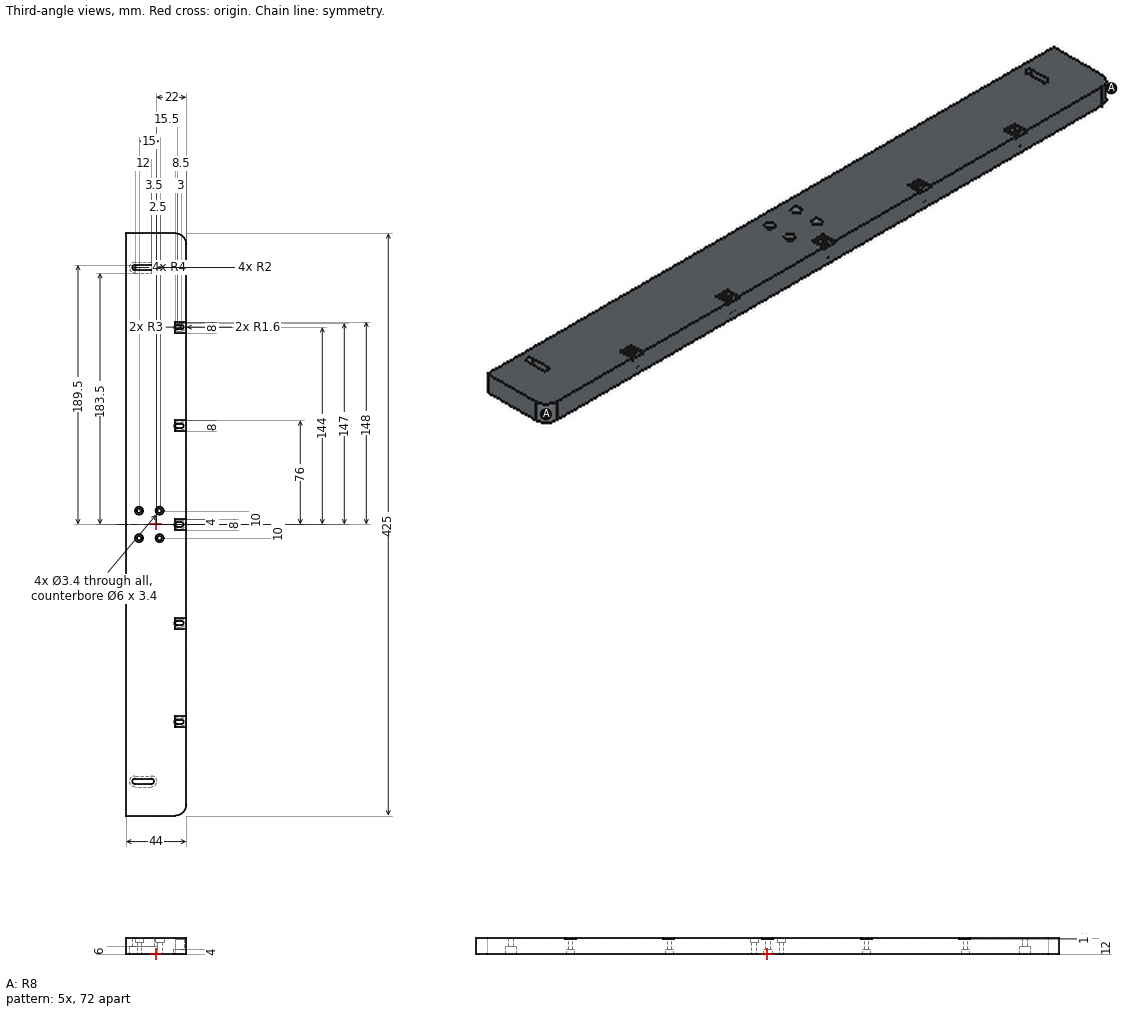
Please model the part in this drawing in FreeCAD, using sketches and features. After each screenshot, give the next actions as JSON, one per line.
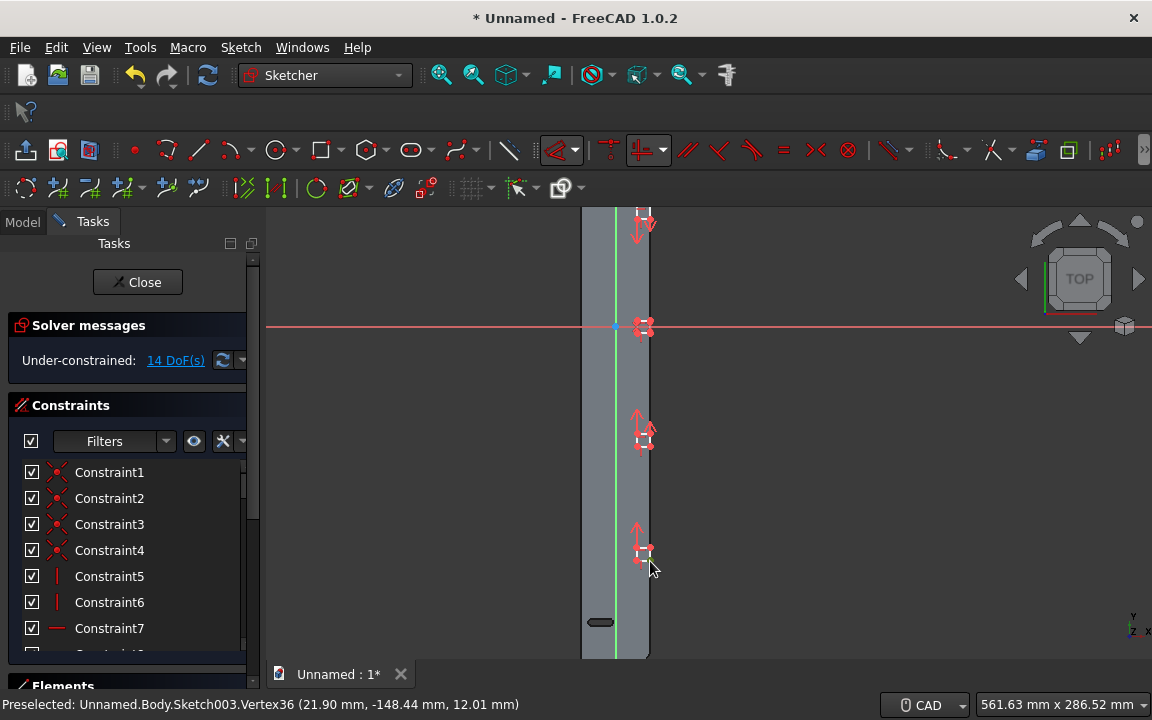
{"action": "left_click", "coordinate": [344, 327]}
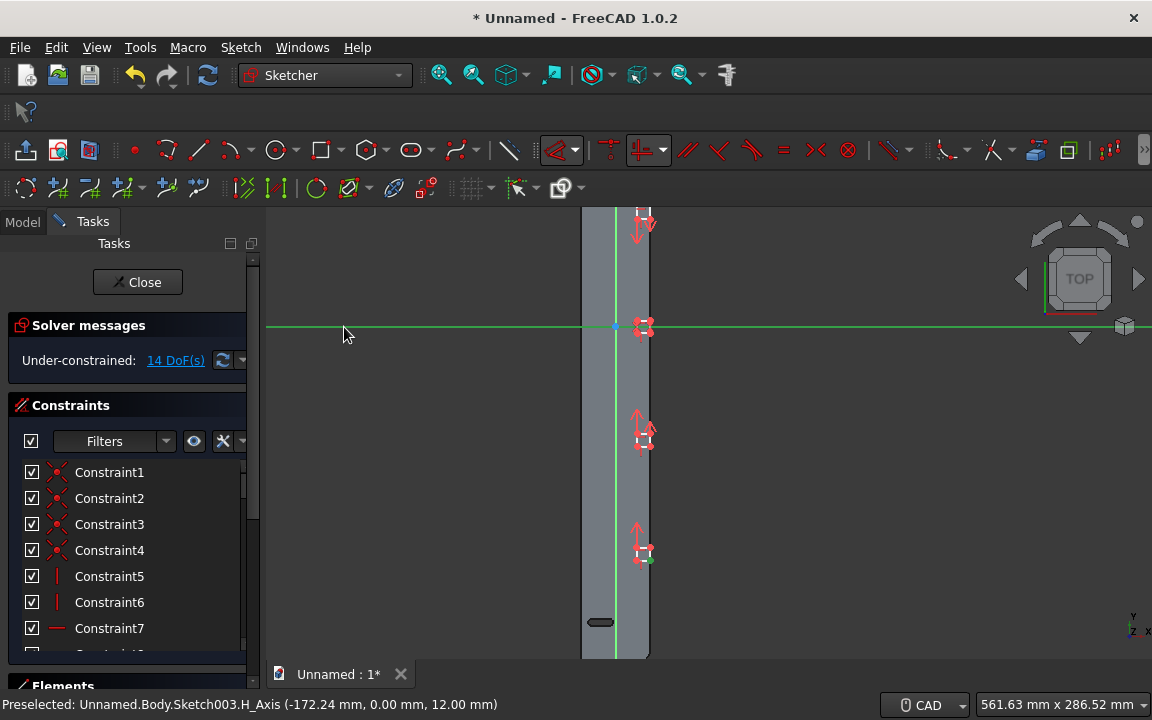
{"action": "key", "text": "s"}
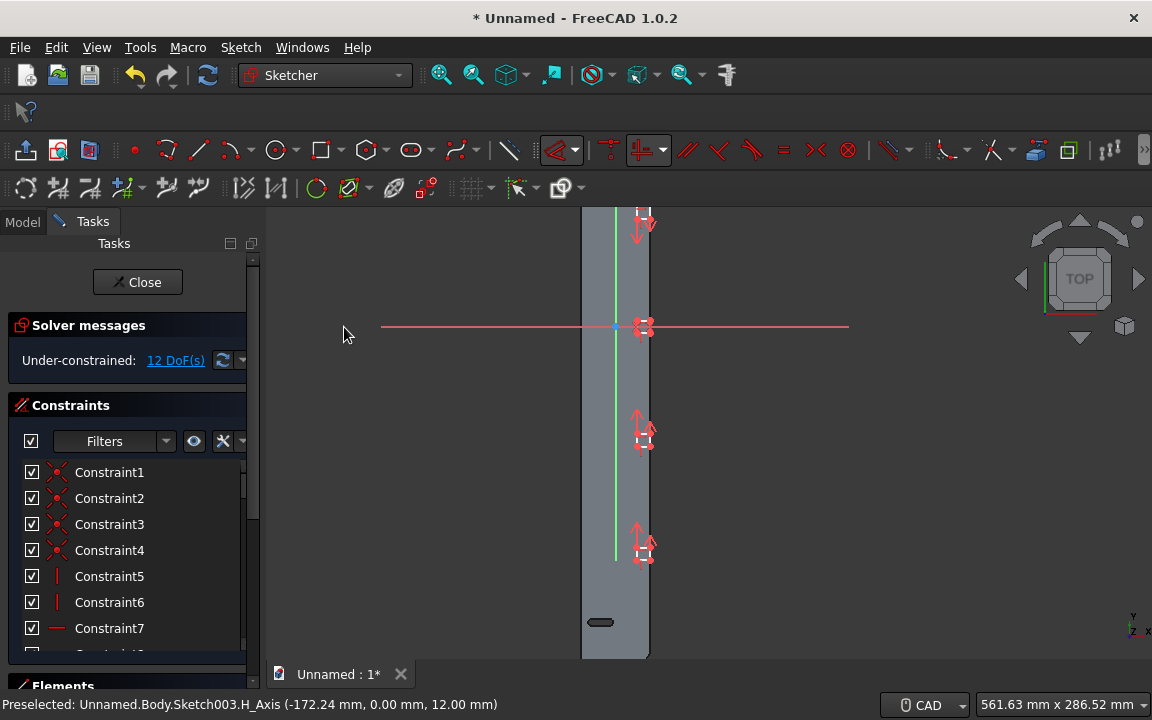
{"action": "scroll", "coordinate": [650, 562], "scroll_direction": "down", "scroll_amount": 3}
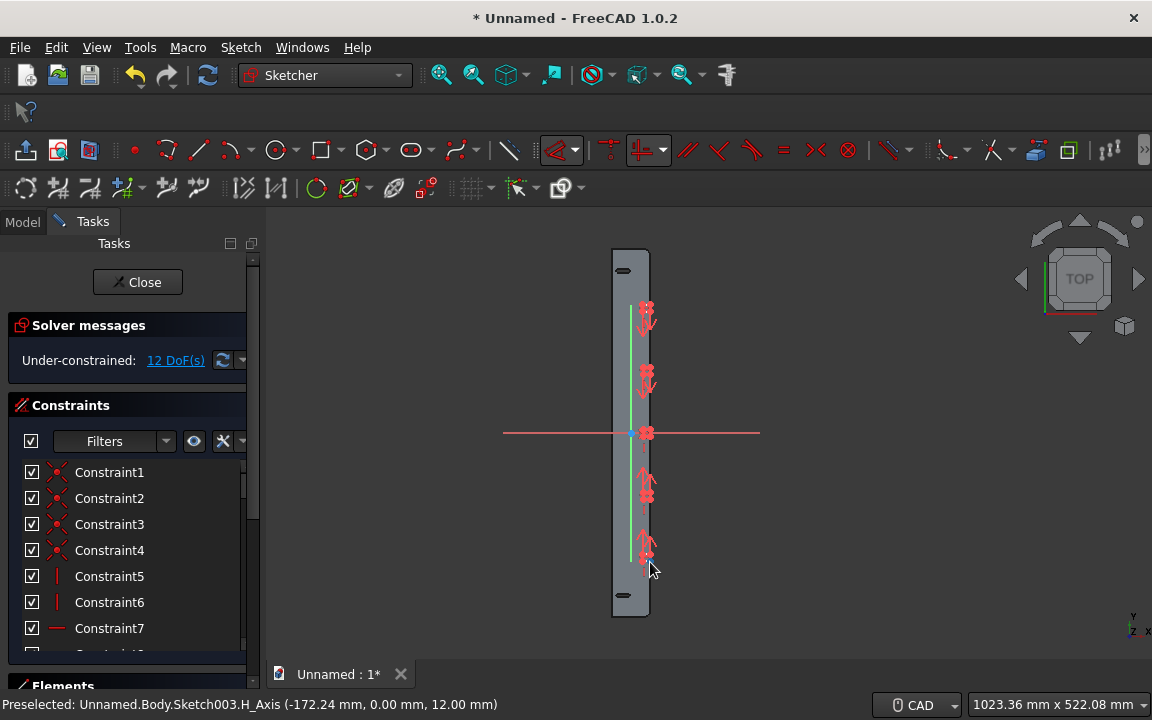
{"action": "scroll", "coordinate": [643, 308], "scroll_direction": "up", "scroll_amount": 9}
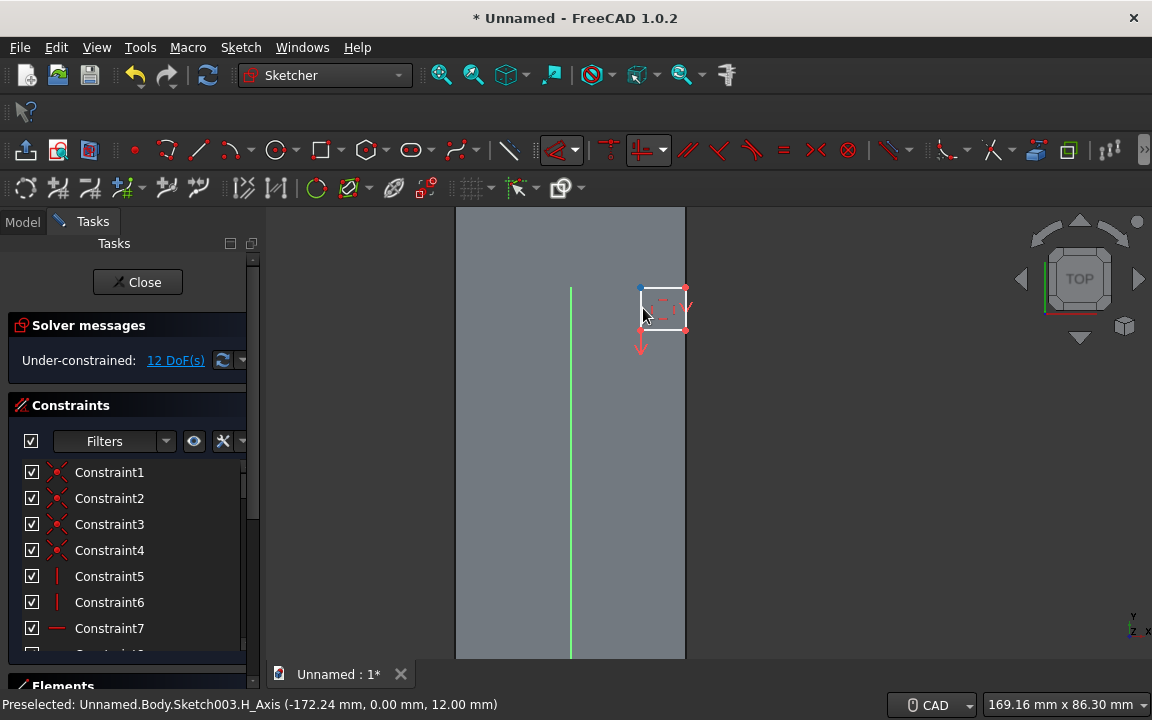
{"action": "left_click", "coordinate": [641, 309]}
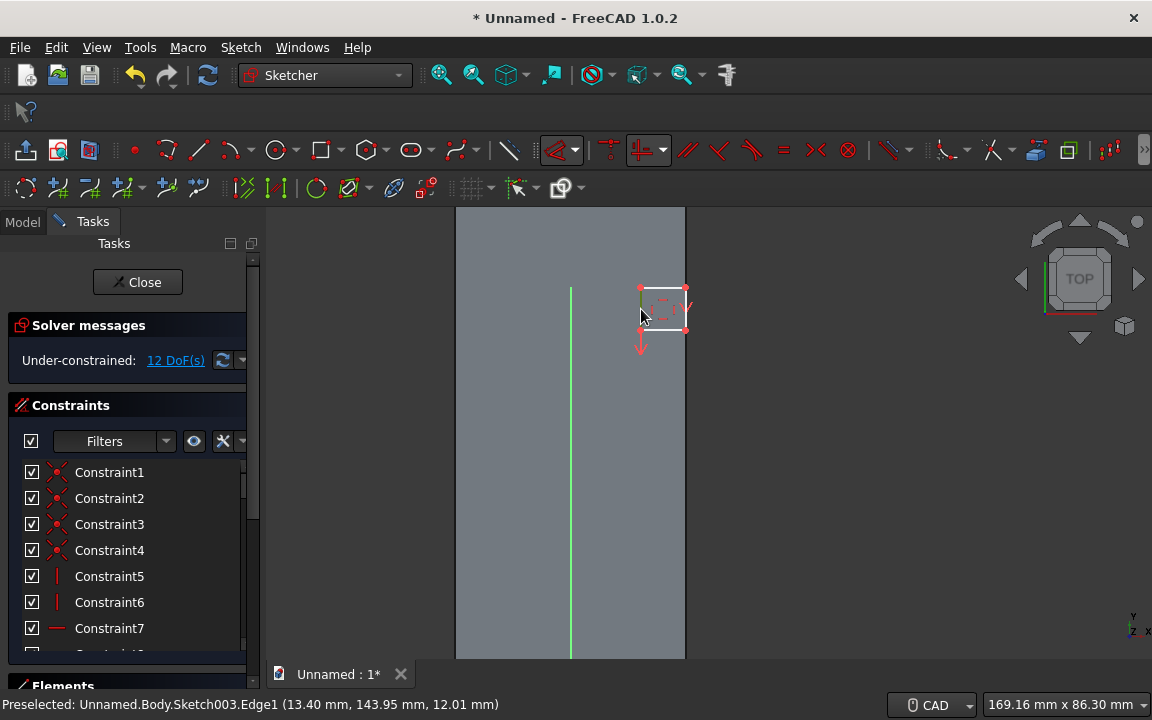
{"action": "key", "text": "i"}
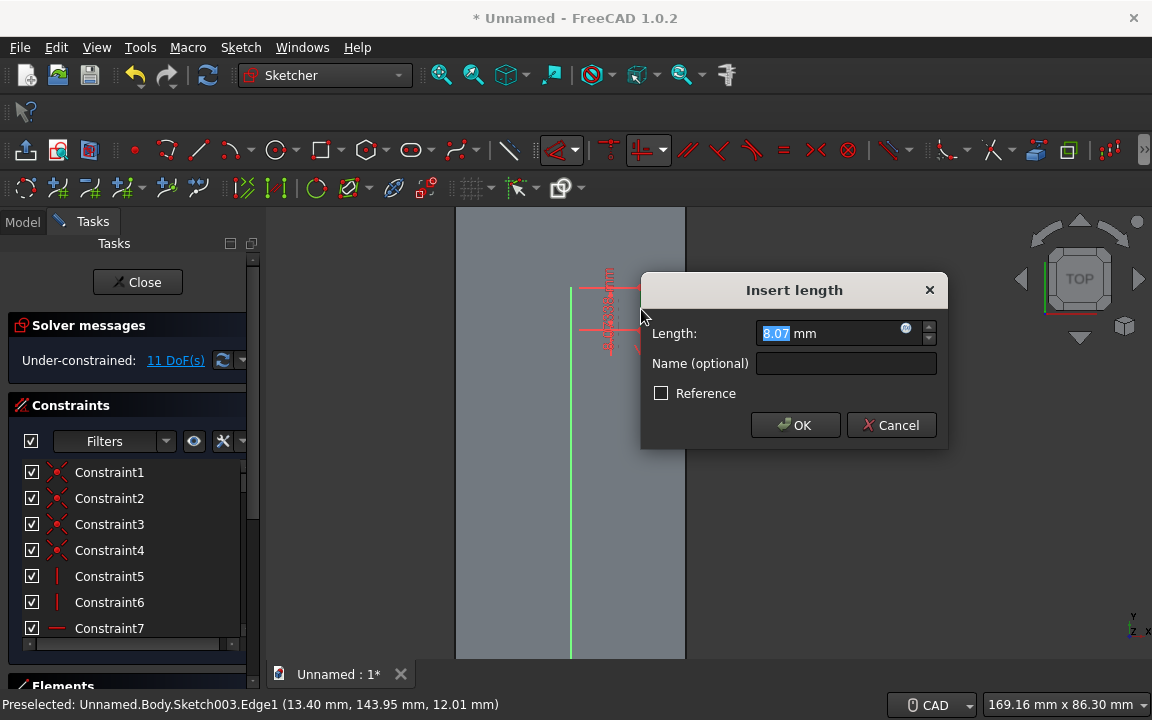
{"action": "type", "text": "8"}
{"action": "key", "text": "Return"}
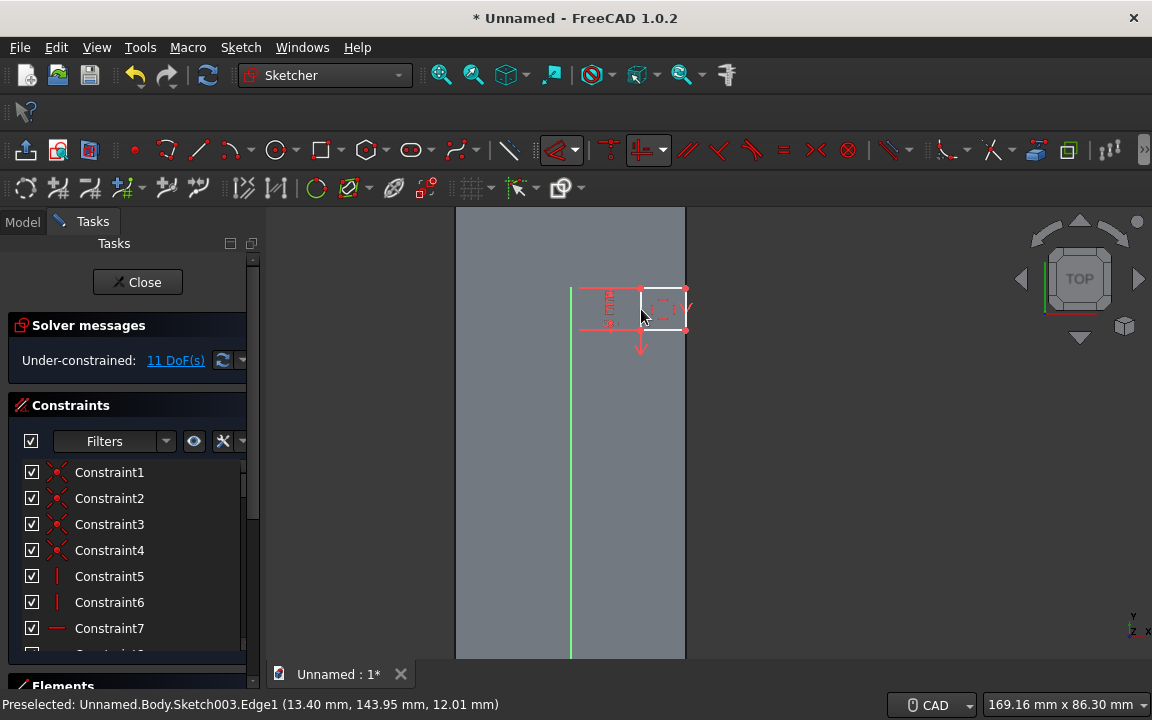
{"action": "scroll", "coordinate": [643, 308], "scroll_direction": "down", "scroll_amount": 9}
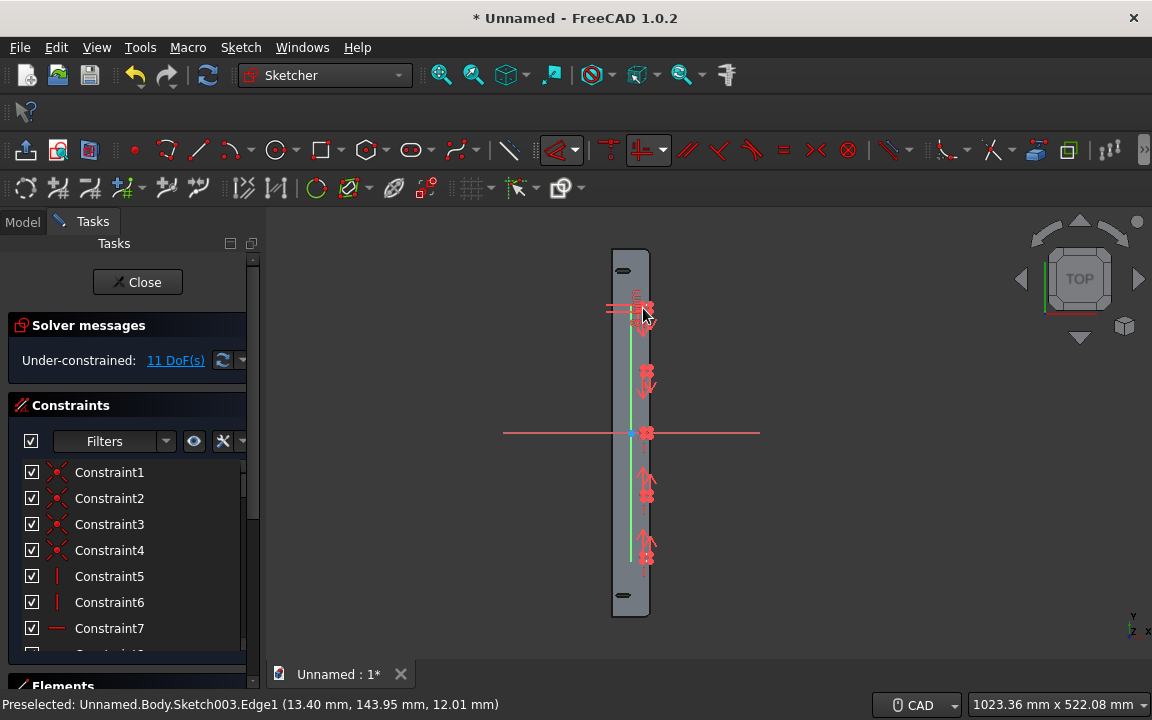
{"action": "scroll", "coordinate": [643, 369], "scroll_direction": "up", "scroll_amount": 10}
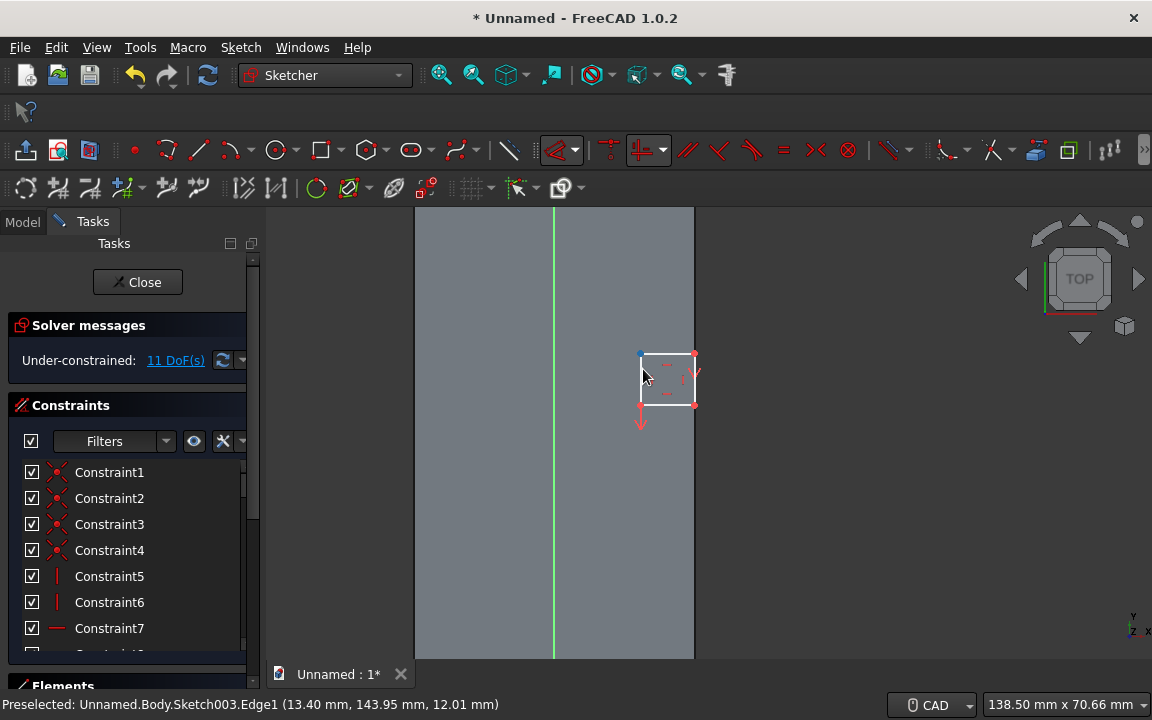
{"action": "left_click", "coordinate": [641, 369]}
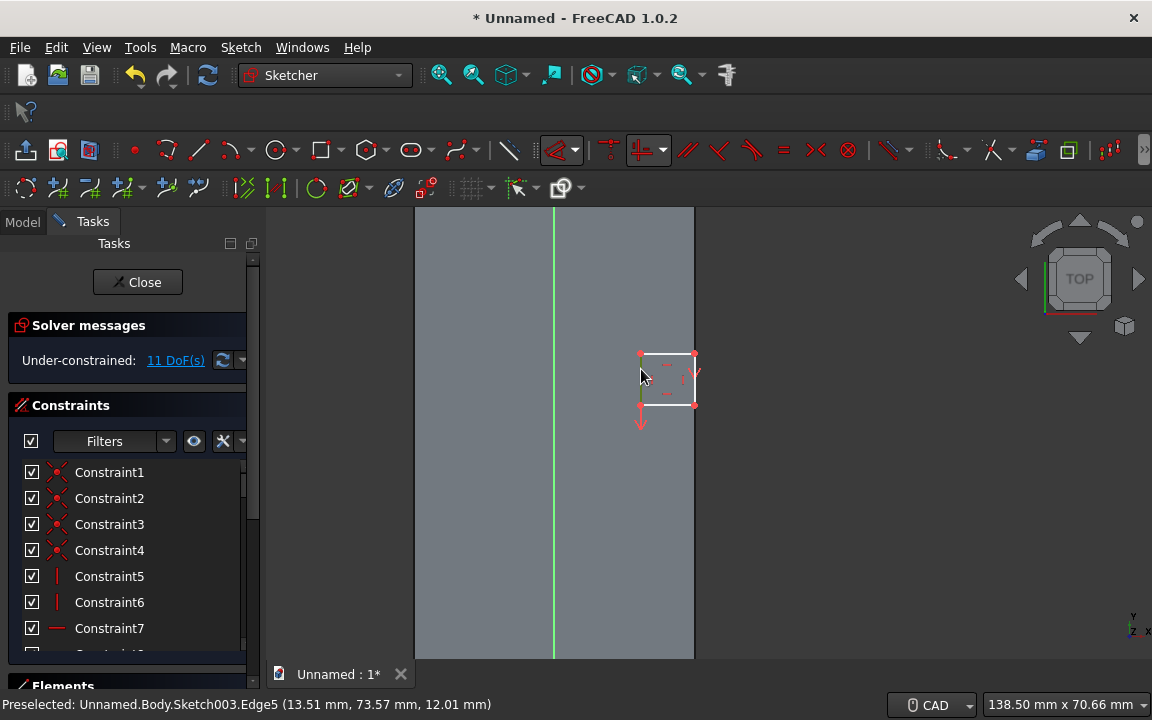
{"action": "key", "text": "i"}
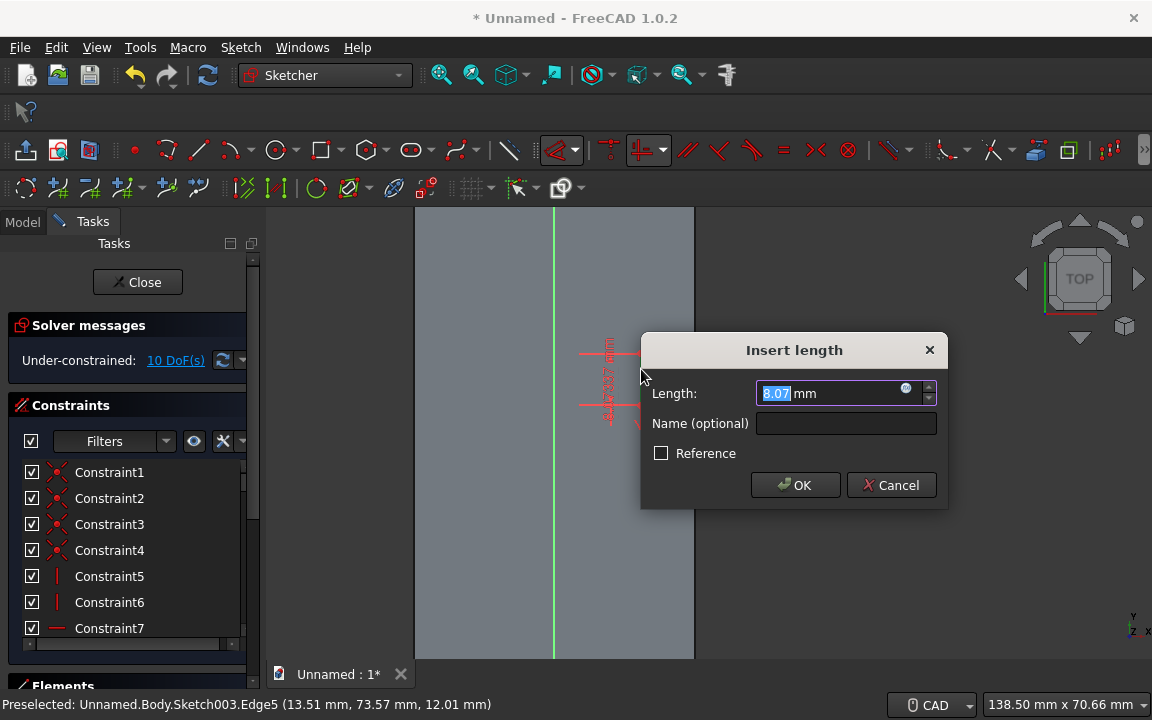
{"action": "type", "text": "8"}
{"action": "key", "text": "Return"}